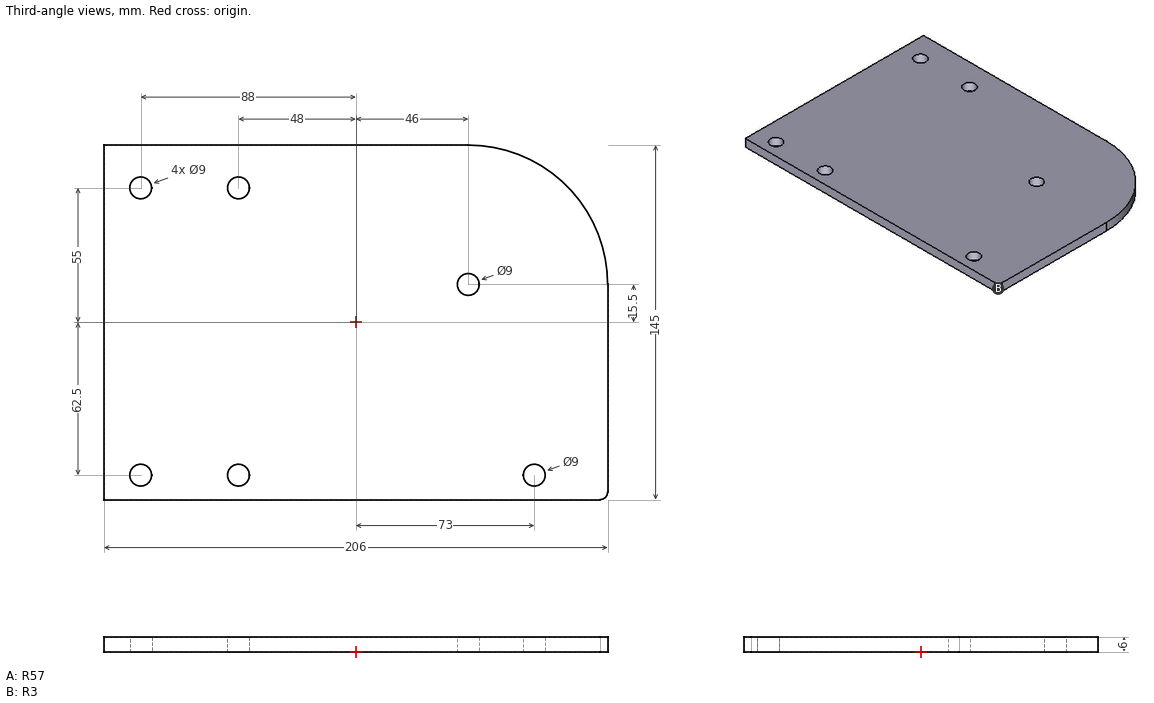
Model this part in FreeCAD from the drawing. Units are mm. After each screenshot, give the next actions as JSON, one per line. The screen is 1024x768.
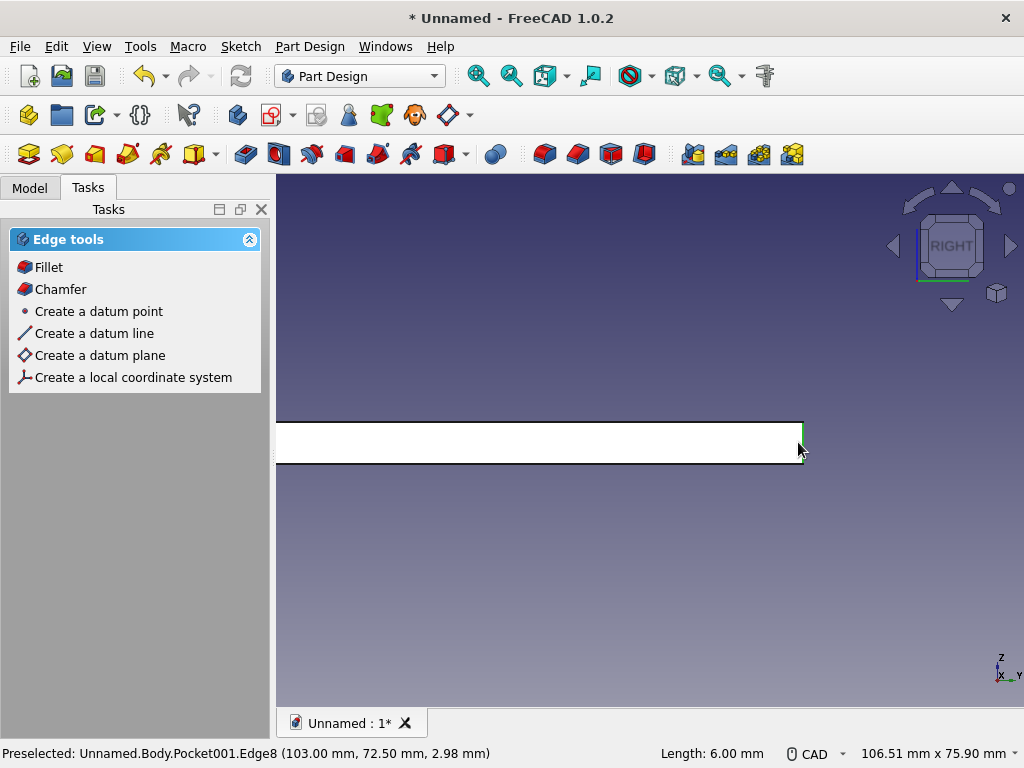
{"action": "left_click", "coordinate": [545, 154]}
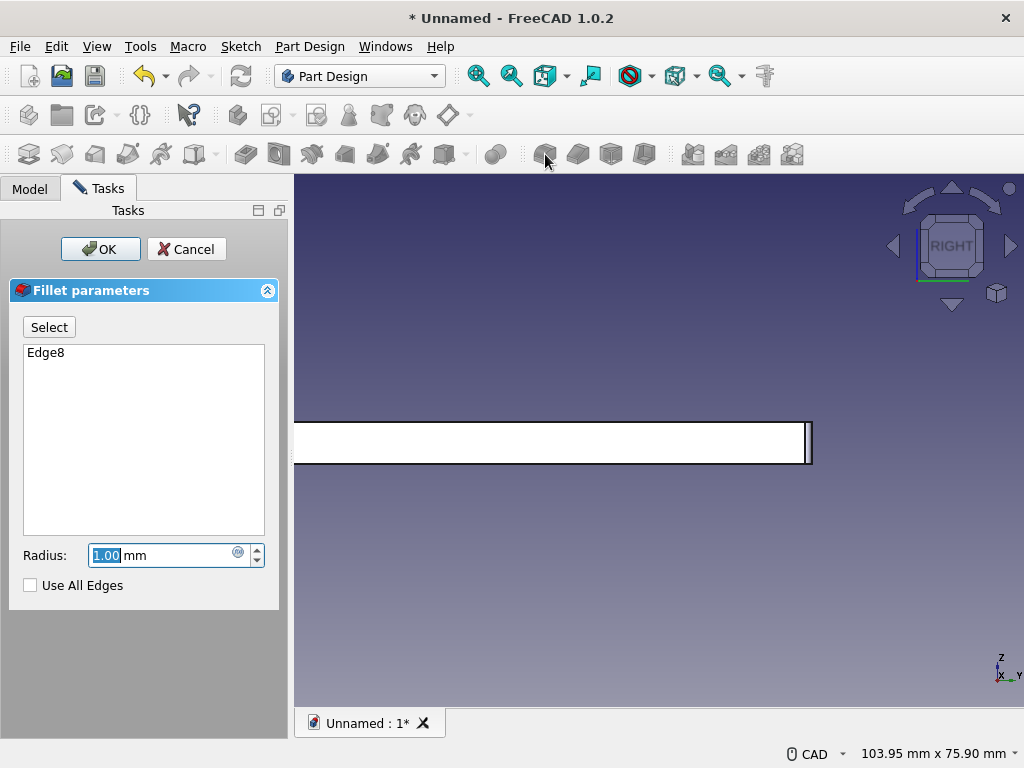
{"action": "type", "text": "57"}
{"action": "key", "text": "Tab"}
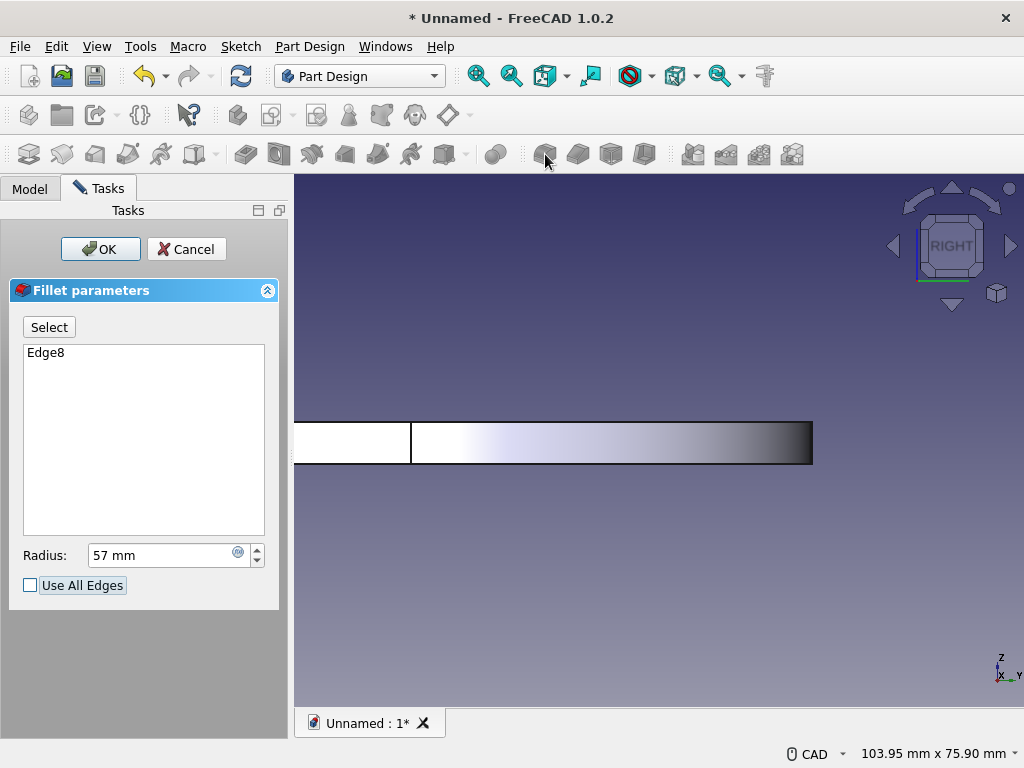
{"action": "left_click", "coordinate": [101, 249]}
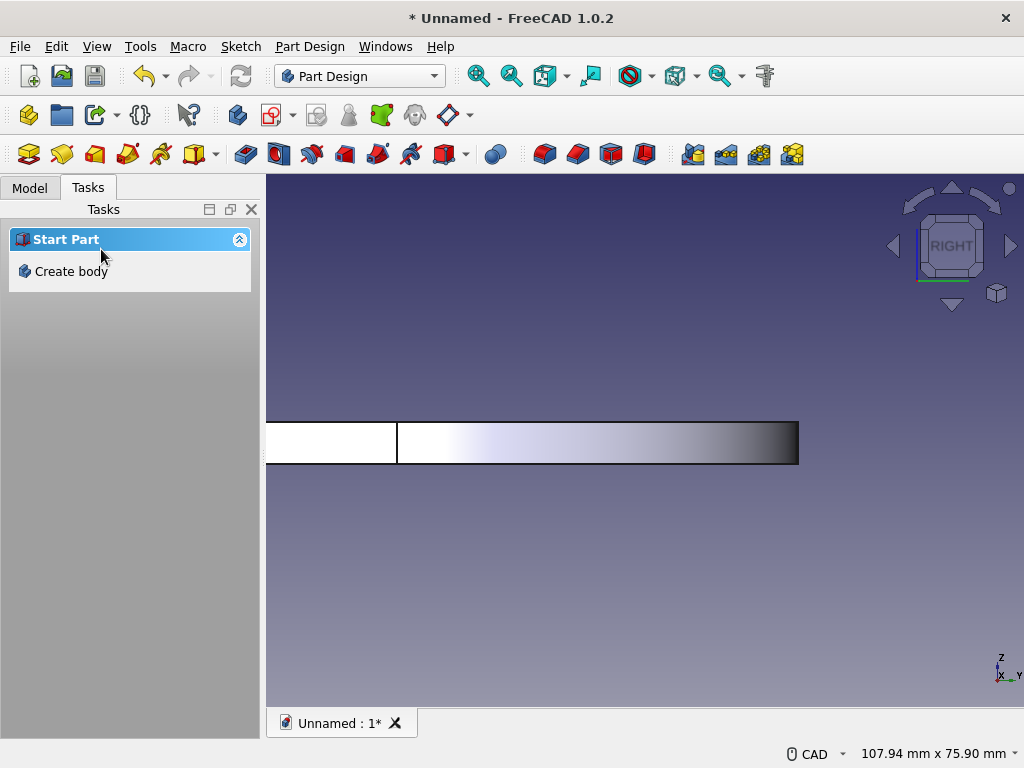
{"action": "left_click", "coordinate": [479, 76]}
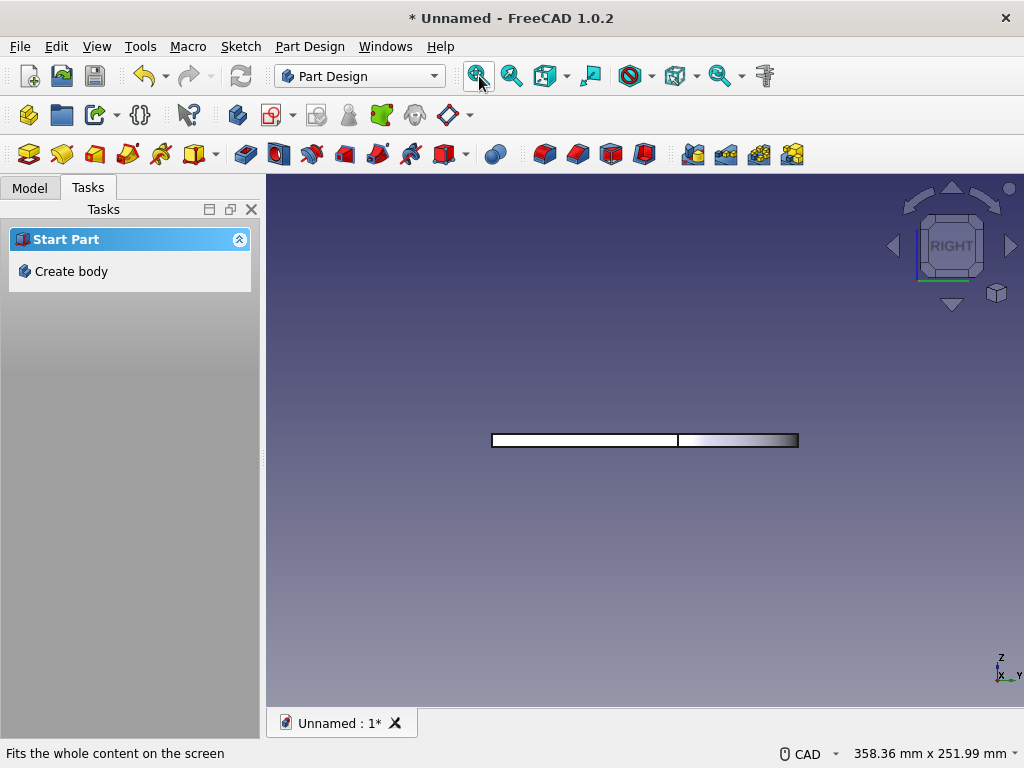
{"action": "key", "text": "5"}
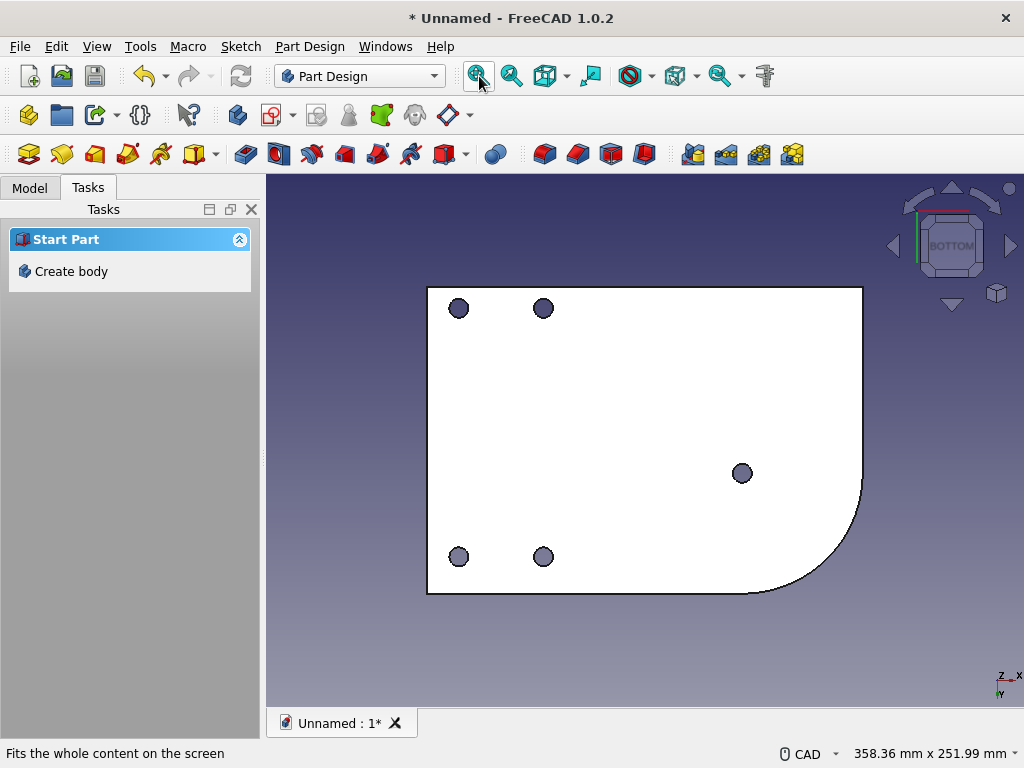
{"action": "left_click", "coordinate": [583, 439]}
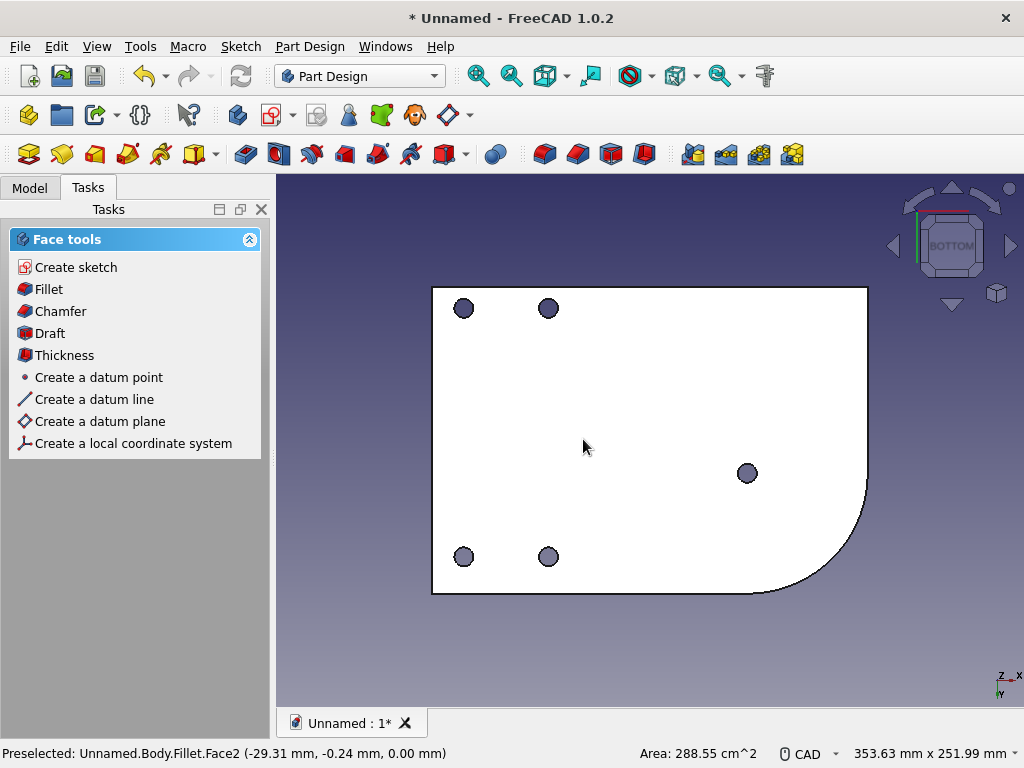
{"action": "left_click", "coordinate": [270, 116]}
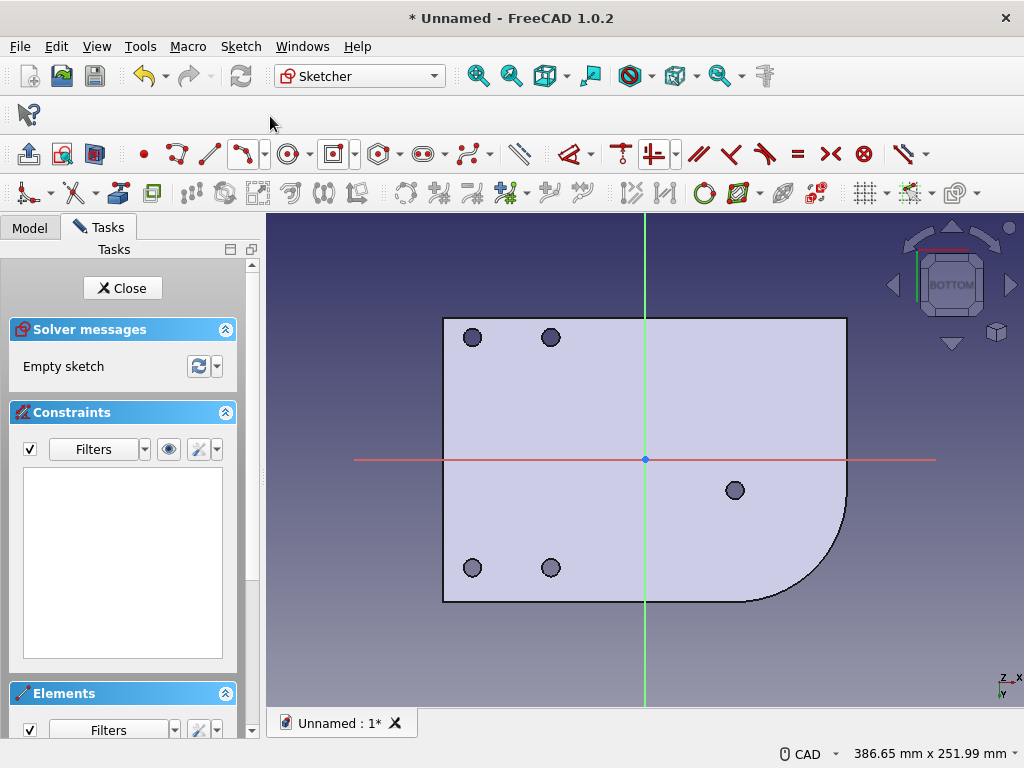
{"action": "scroll", "coordinate": [802, 330], "scroll_direction": "up", "scroll_amount": 14}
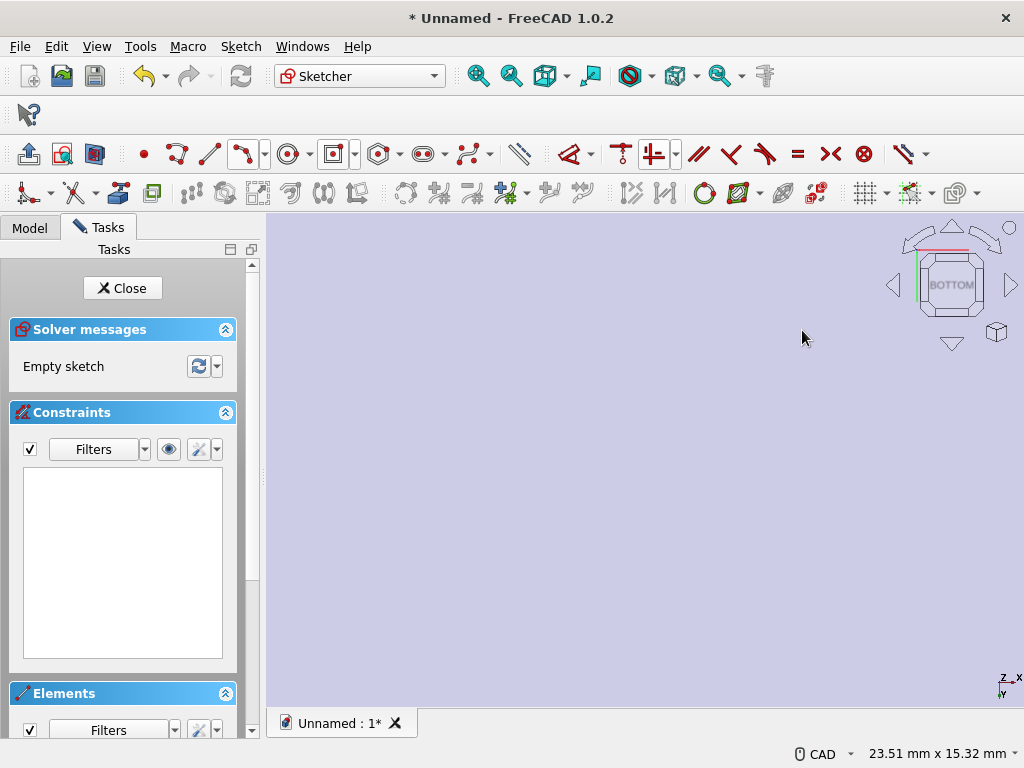
{"action": "key", "text": "g c"}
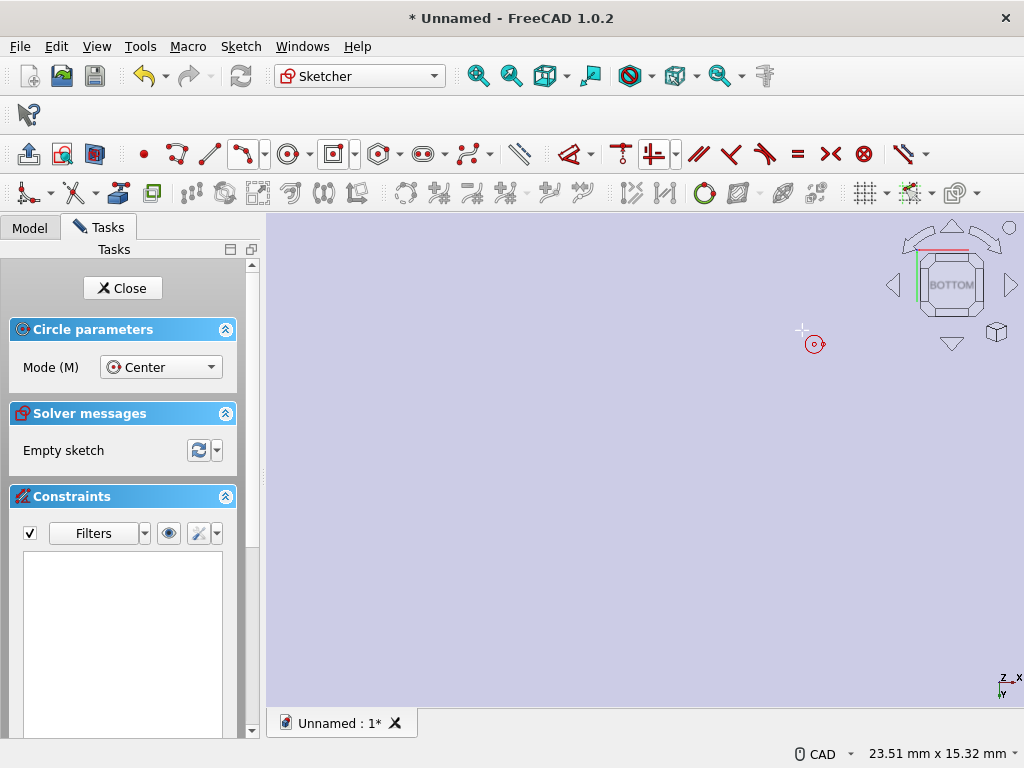
{"action": "left_click", "coordinate": [563, 449]}
{"action": "mouse_move", "coordinate": [665, 347]}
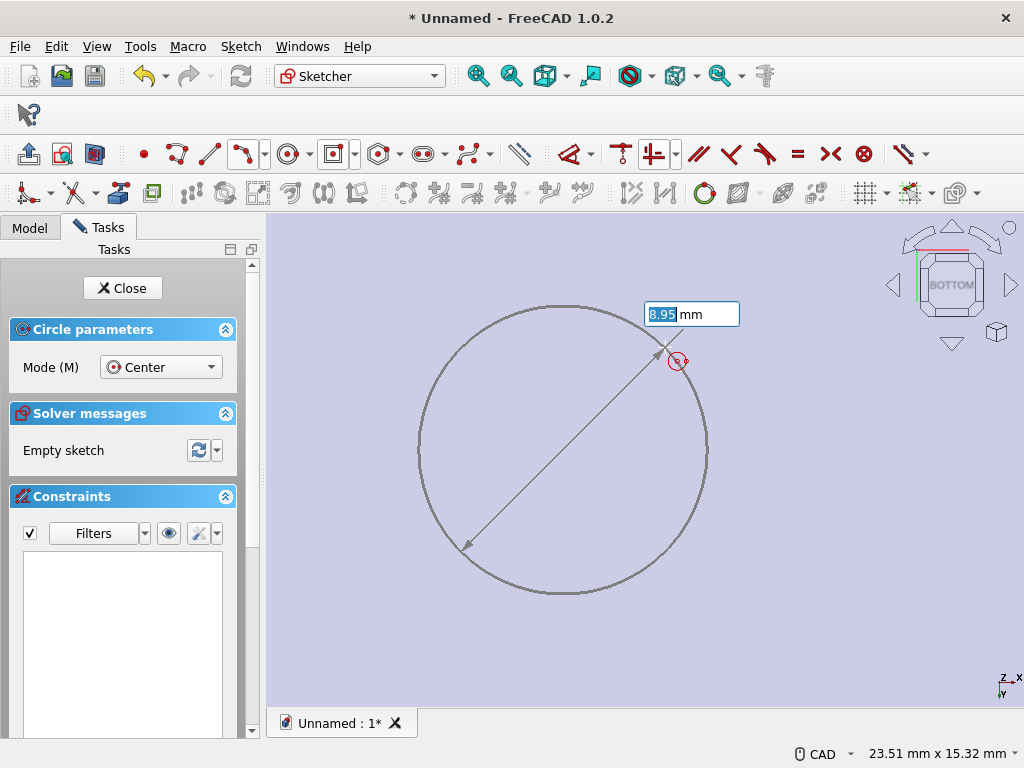
{"action": "type", "text": "9"}
{"action": "key", "text": "Return"}
{"action": "key", "text": "Escape"}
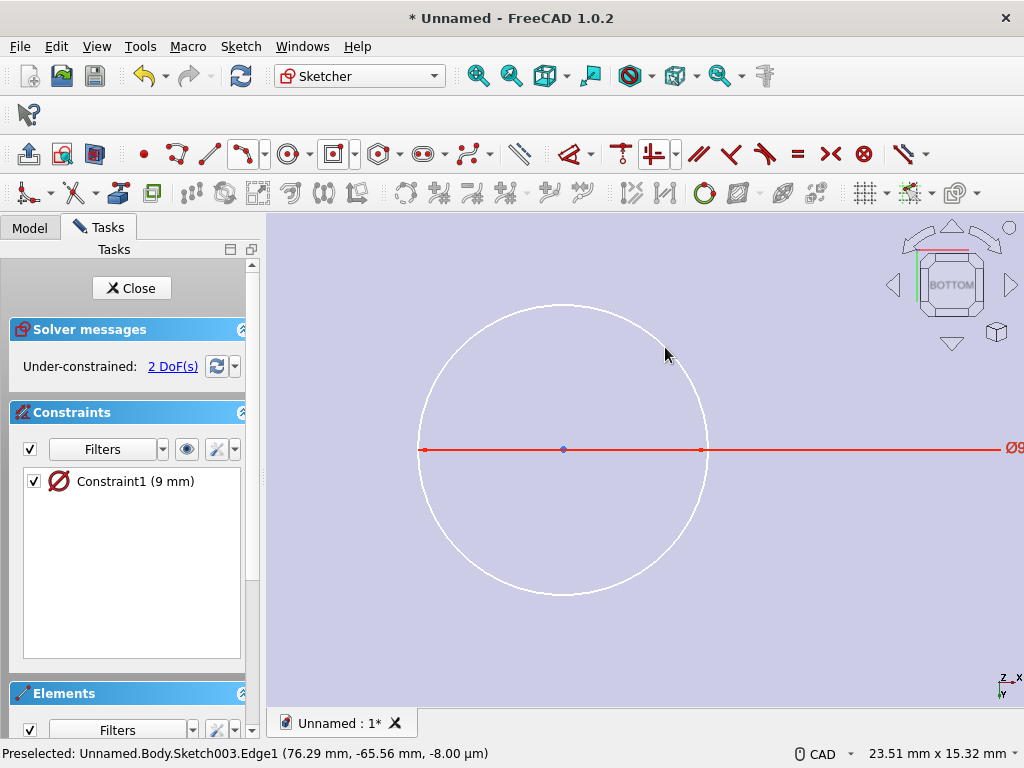
{"action": "left_click", "coordinate": [568, 154]}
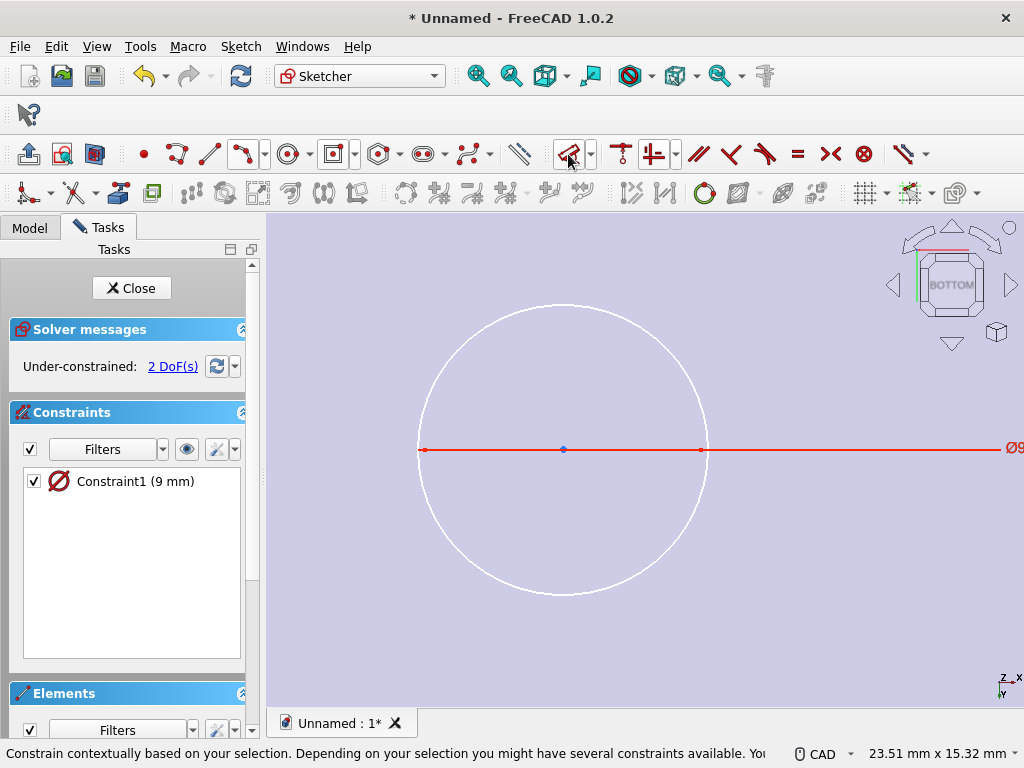
{"action": "left_click", "coordinate": [563, 450]}
{"action": "left_click", "coordinate": [367, 416]}